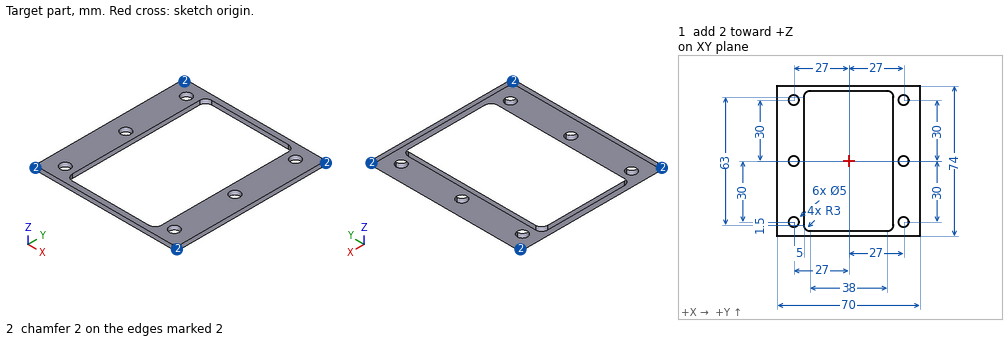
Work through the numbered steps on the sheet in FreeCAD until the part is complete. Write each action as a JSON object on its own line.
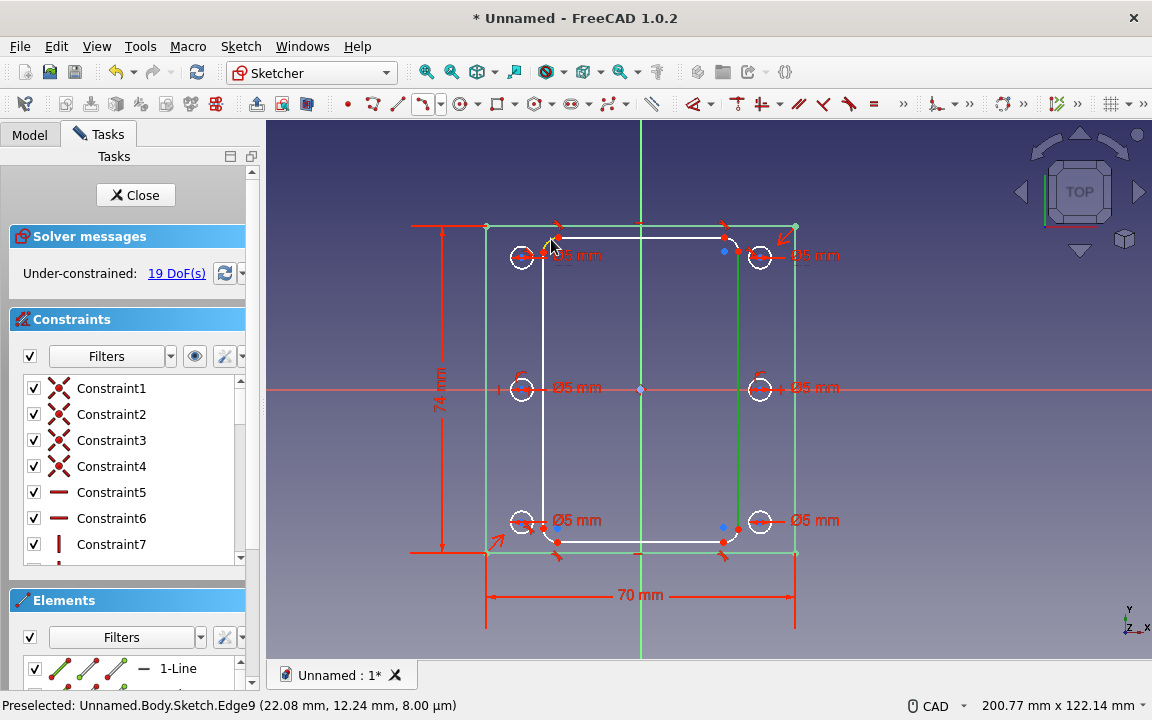
{"action": "scroll", "coordinate": [730, 541], "scroll_direction": "up", "scroll_amount": 4}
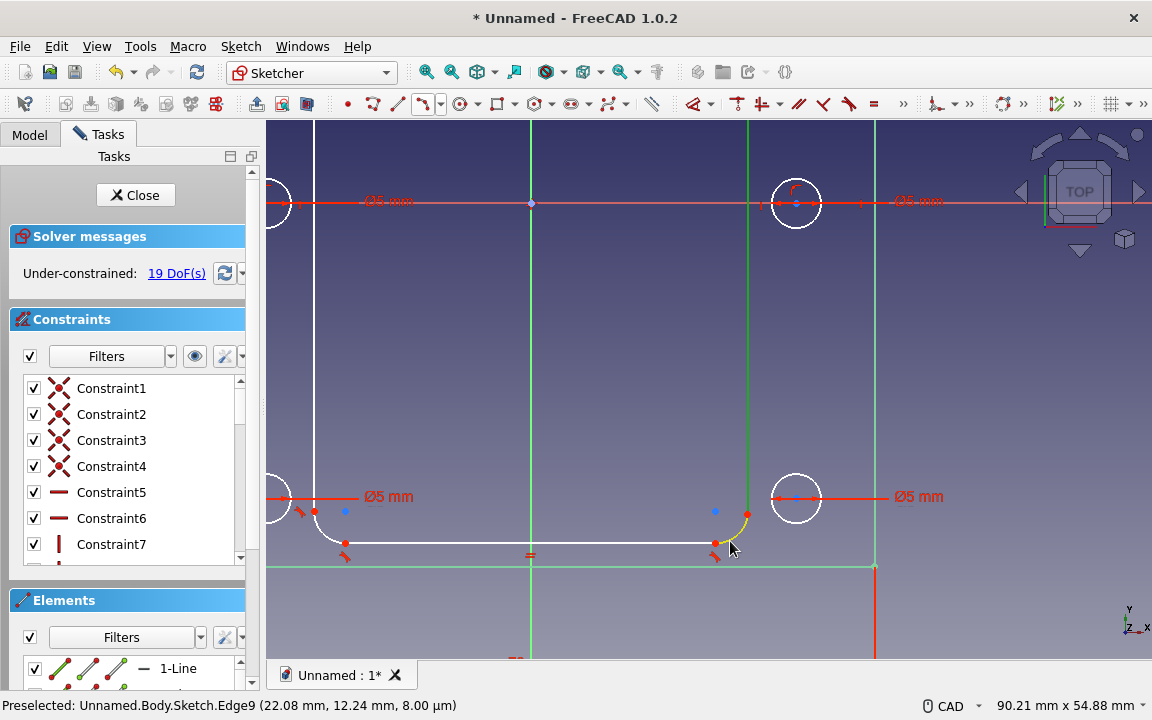
{"action": "left_click", "coordinate": [730, 540]}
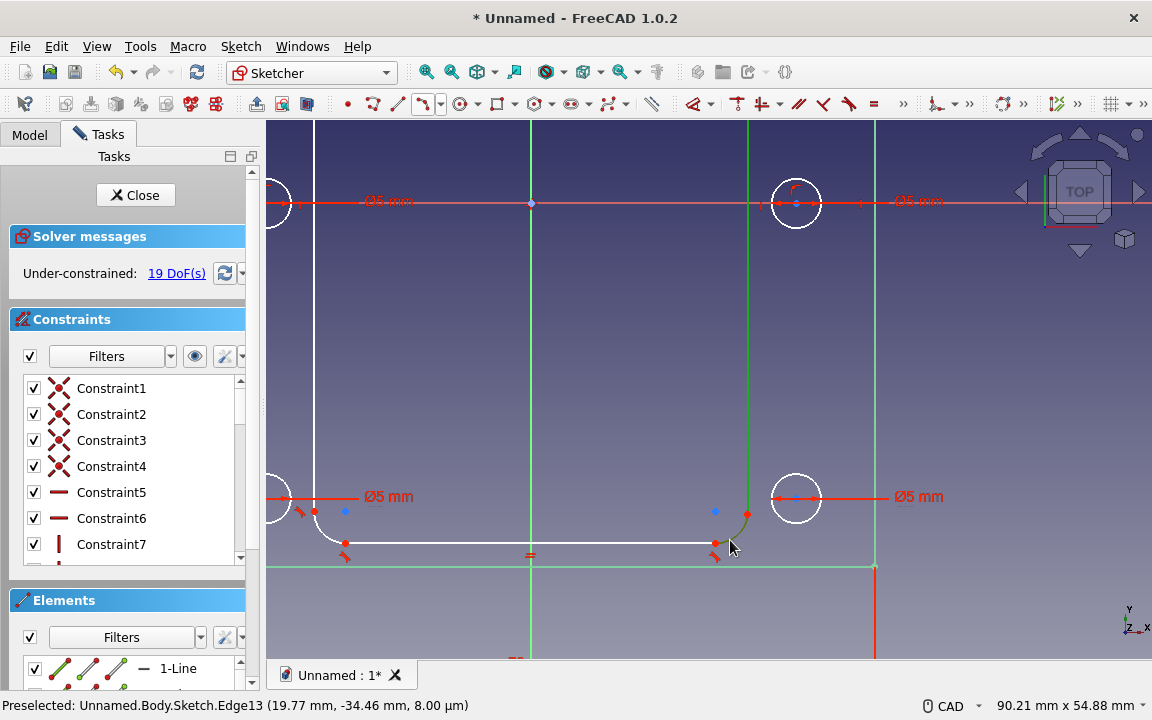
{"action": "left_click", "coordinate": [849, 104]}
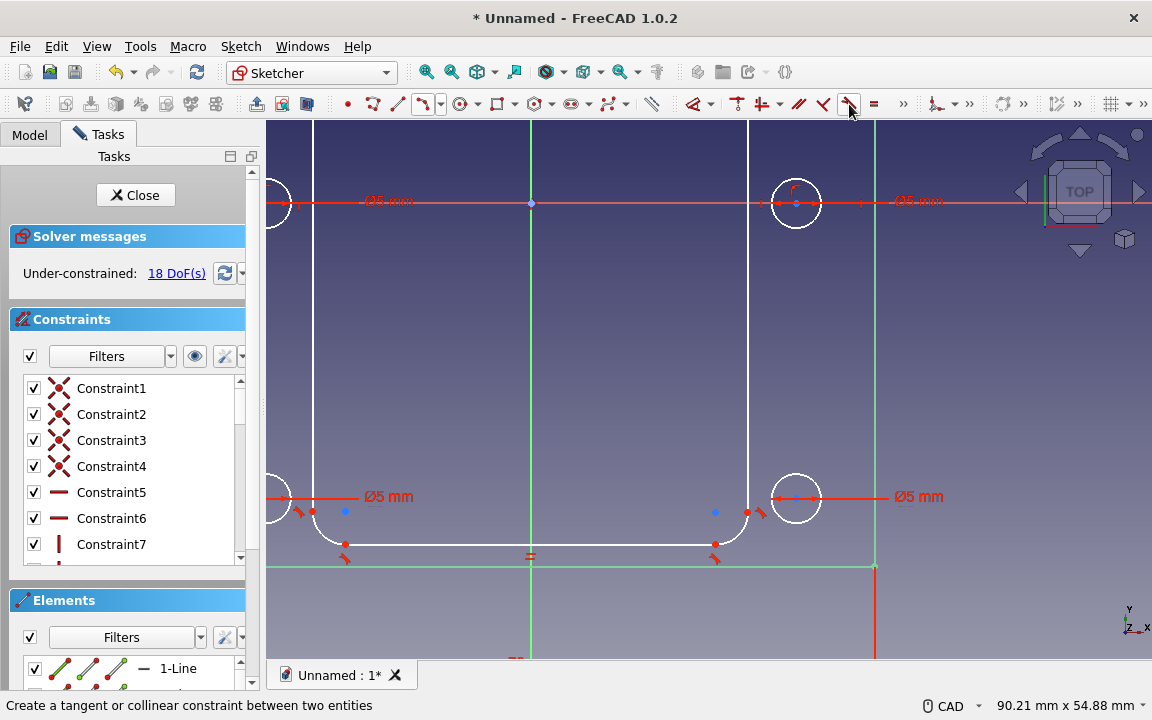
{"action": "left_click", "coordinate": [316, 527]}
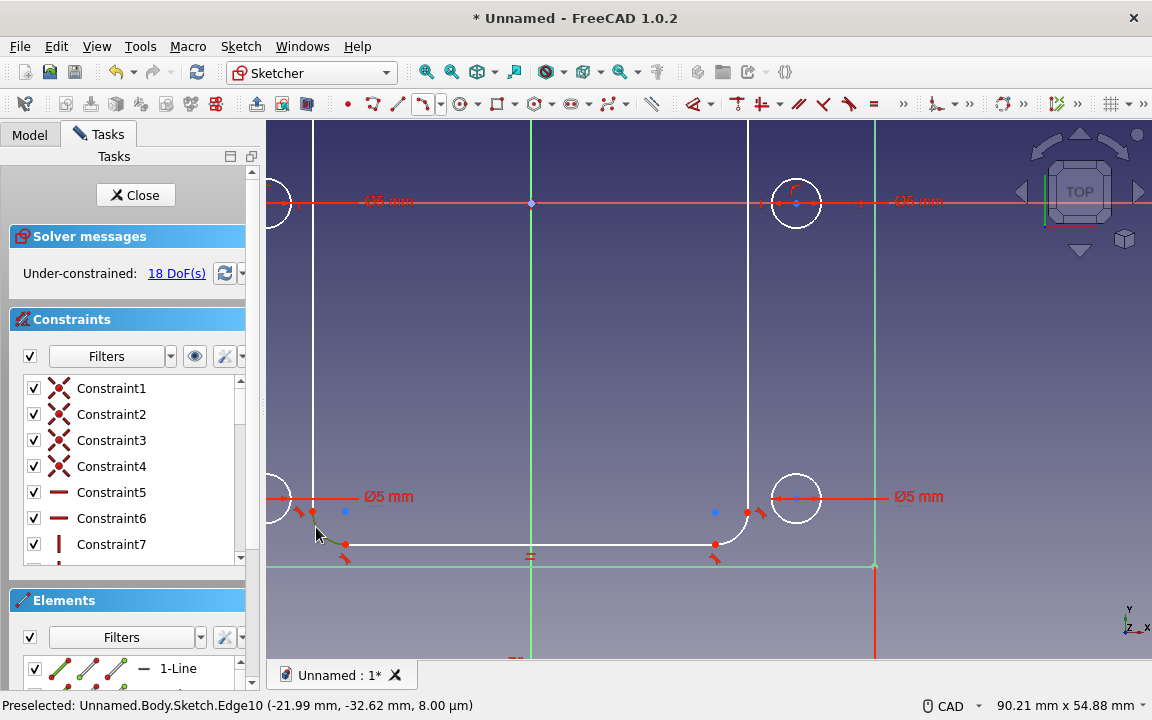
{"action": "scroll", "coordinate": [730, 541], "scroll_direction": "down", "scroll_amount": 4}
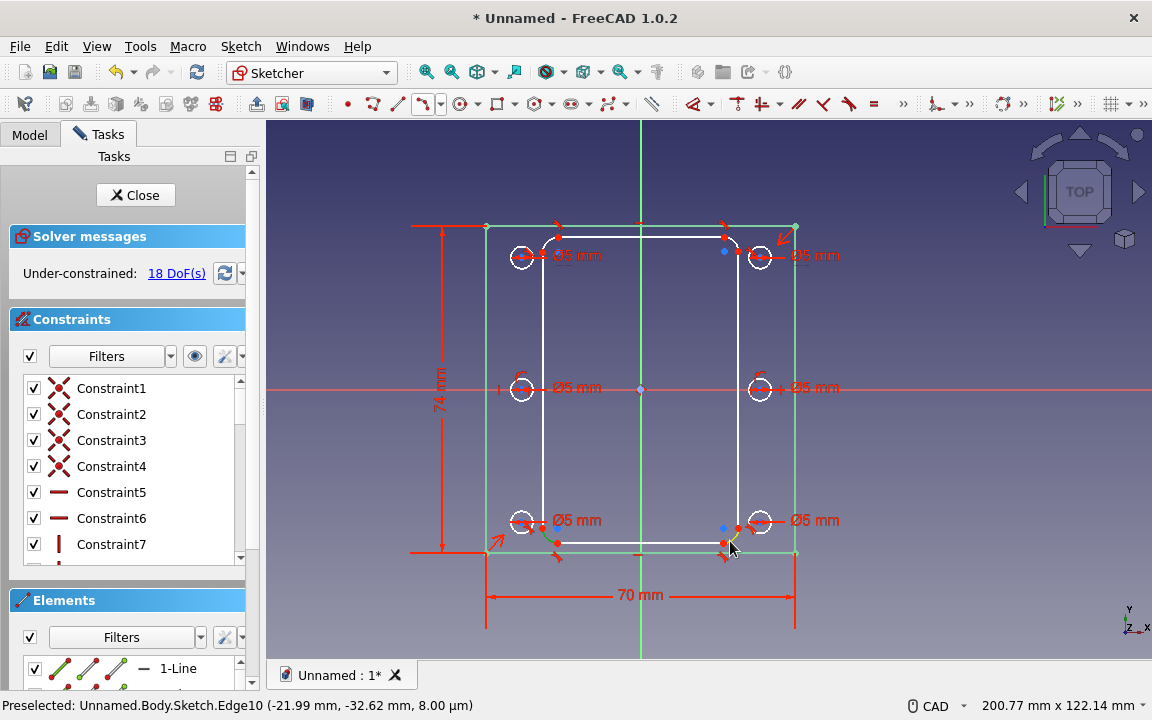
{"action": "scroll", "coordinate": [551, 239], "scroll_direction": "up", "scroll_amount": 4}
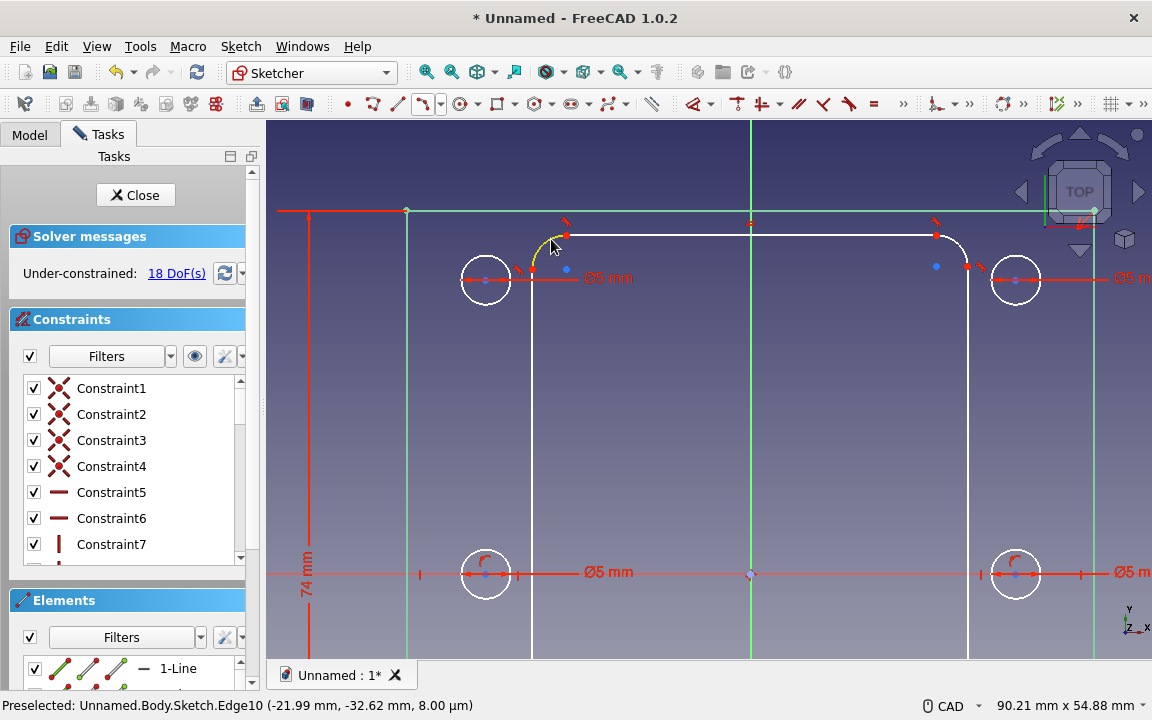
{"action": "left_click", "coordinate": [551, 239]}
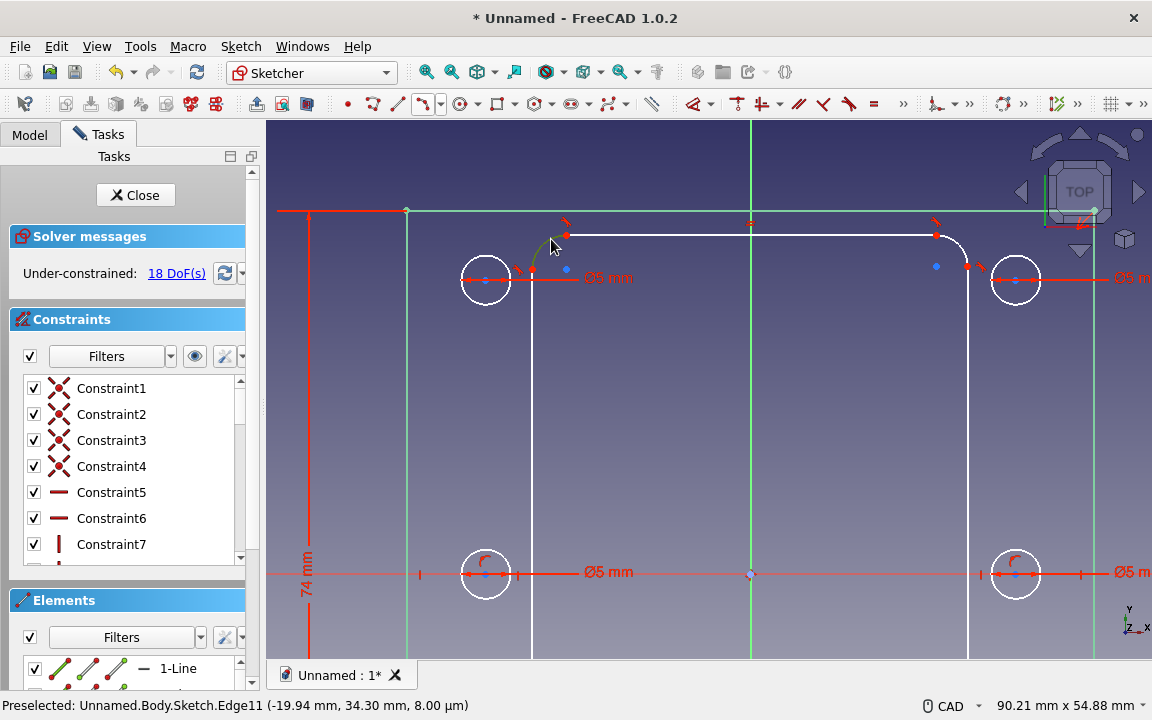
{"action": "left_click", "coordinate": [964, 252]}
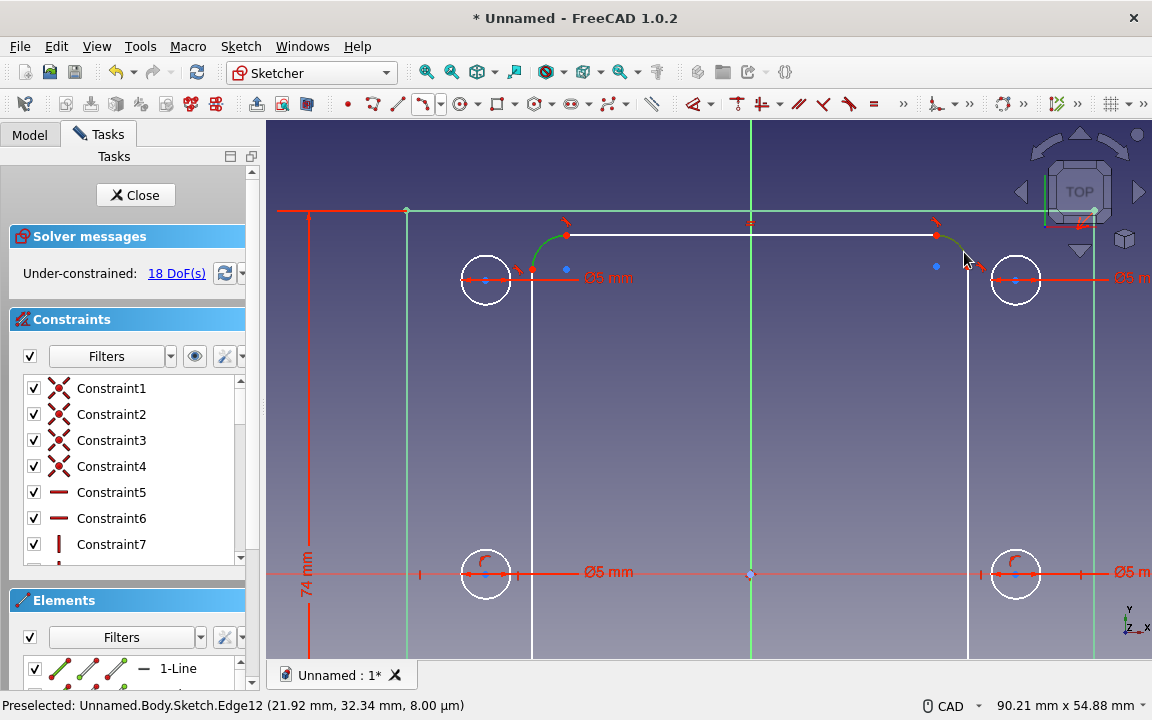
{"action": "scroll", "coordinate": [551, 239], "scroll_direction": "down", "scroll_amount": 4}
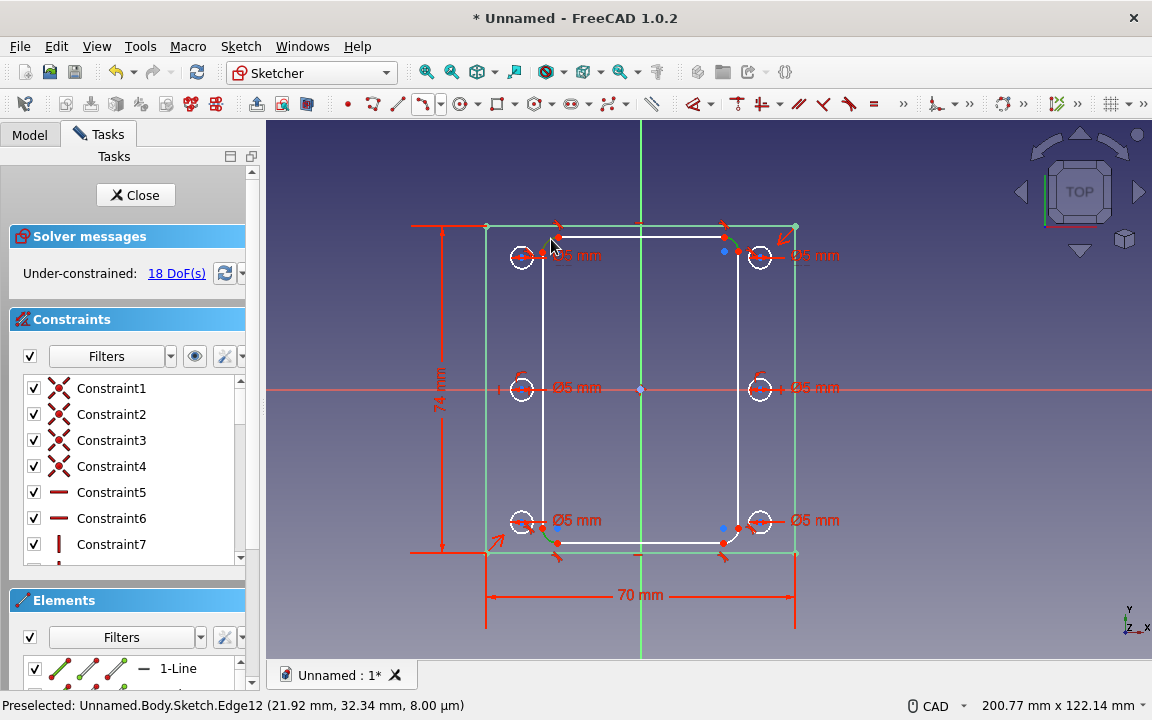
{"action": "scroll", "coordinate": [731, 541], "scroll_direction": "up", "scroll_amount": 4}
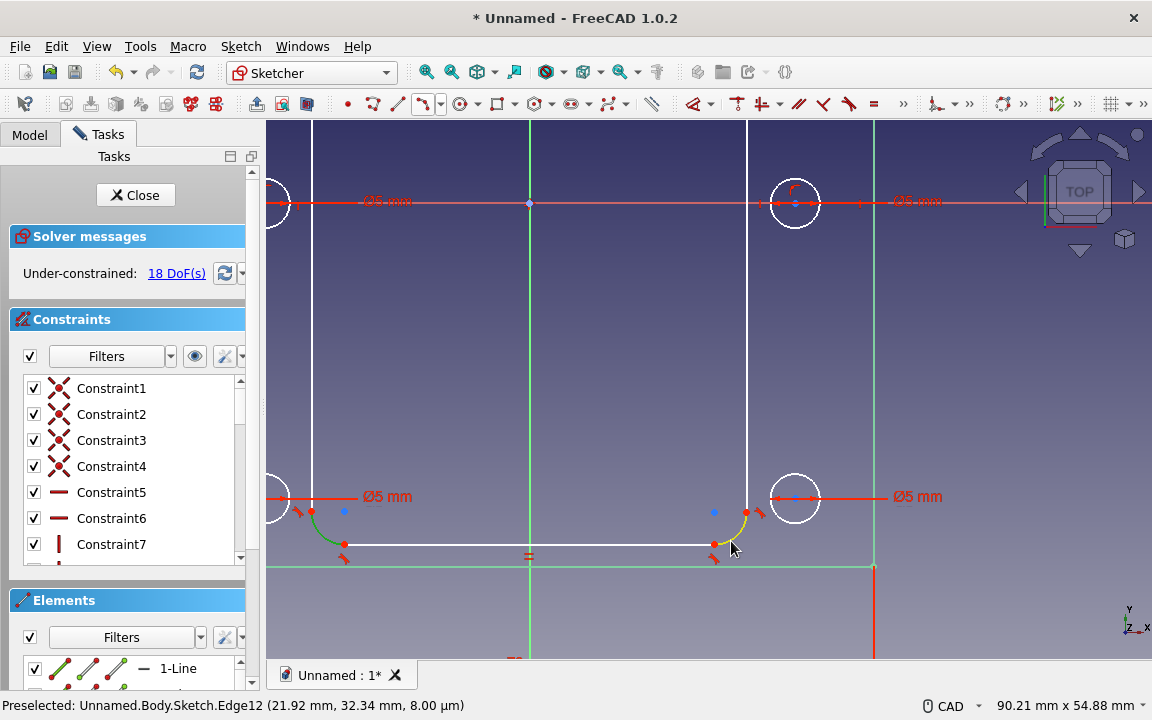
{"action": "left_click", "coordinate": [729, 541]}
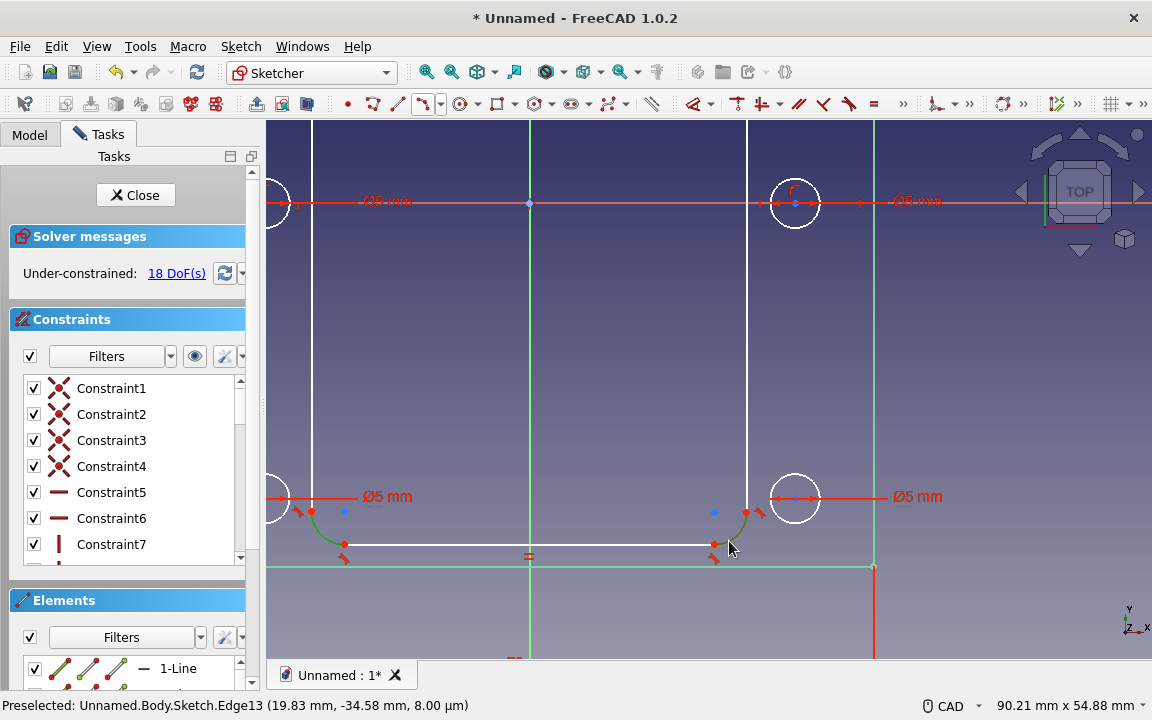
{"action": "left_click", "coordinate": [874, 104]}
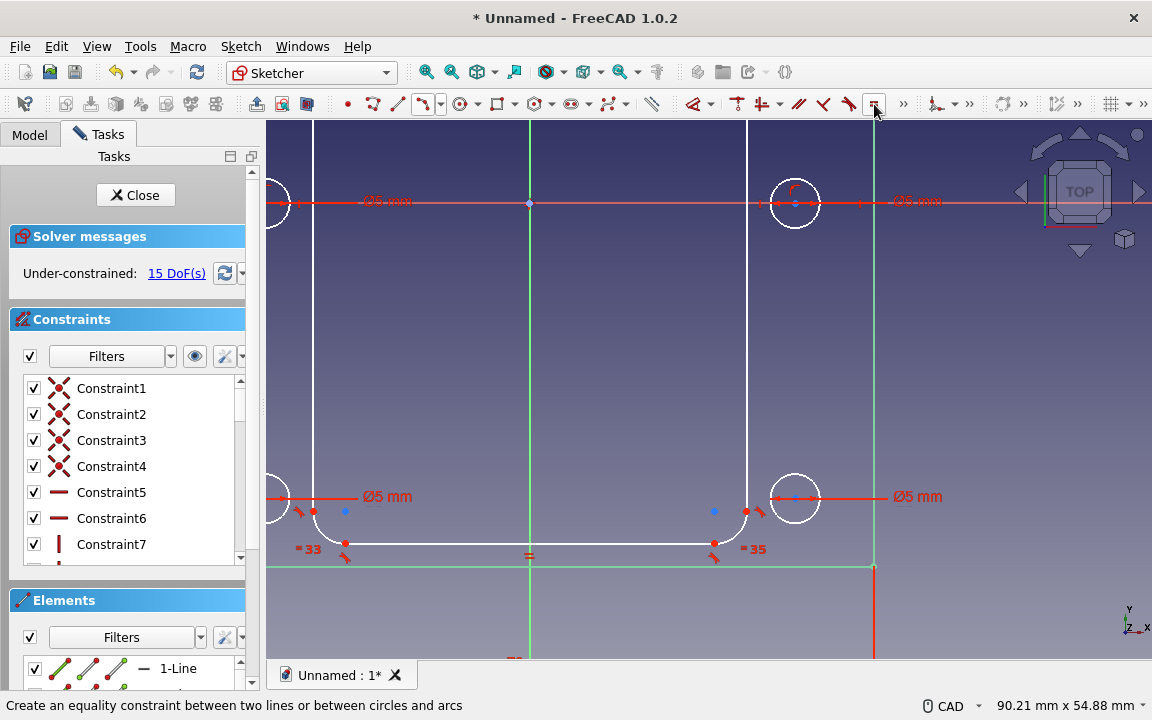
{"action": "scroll", "coordinate": [731, 541], "scroll_direction": "down", "scroll_amount": 4}